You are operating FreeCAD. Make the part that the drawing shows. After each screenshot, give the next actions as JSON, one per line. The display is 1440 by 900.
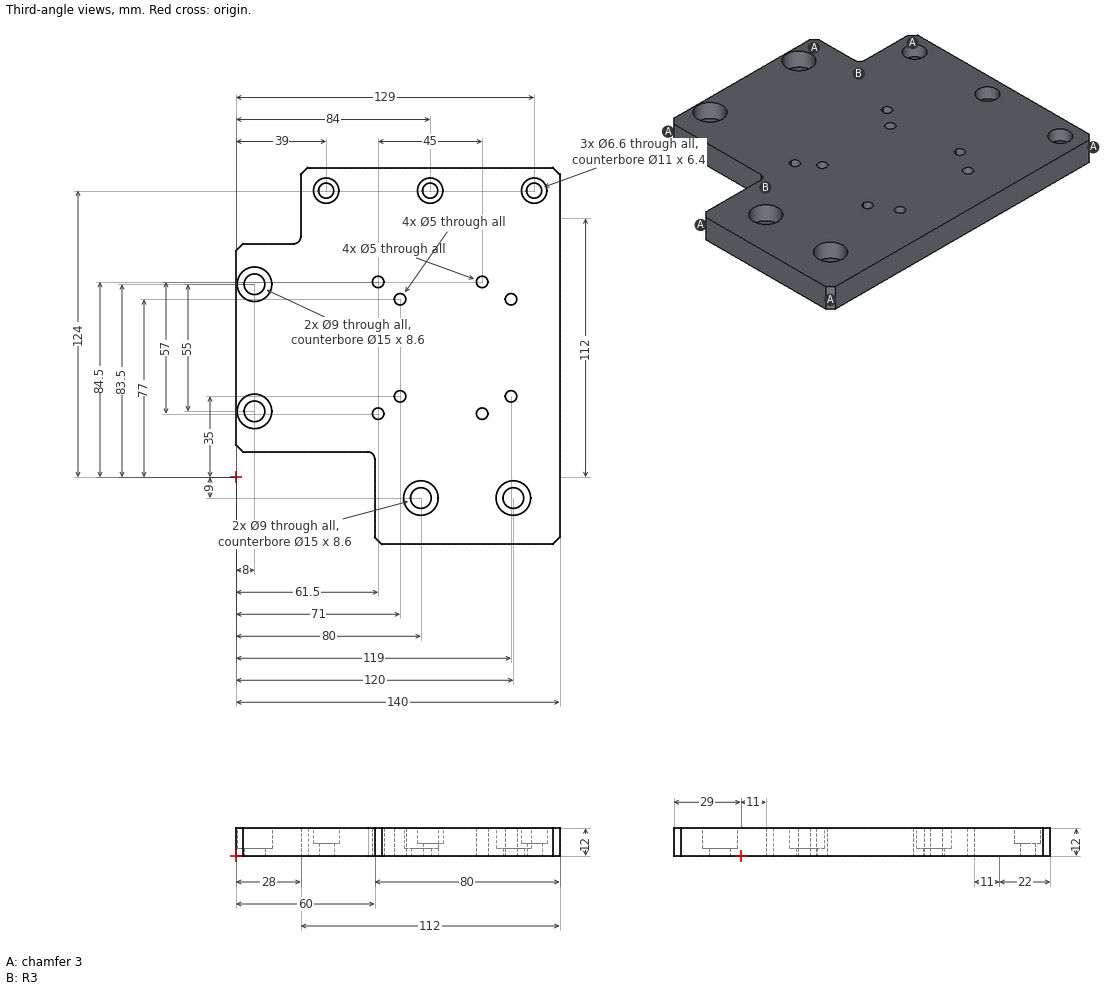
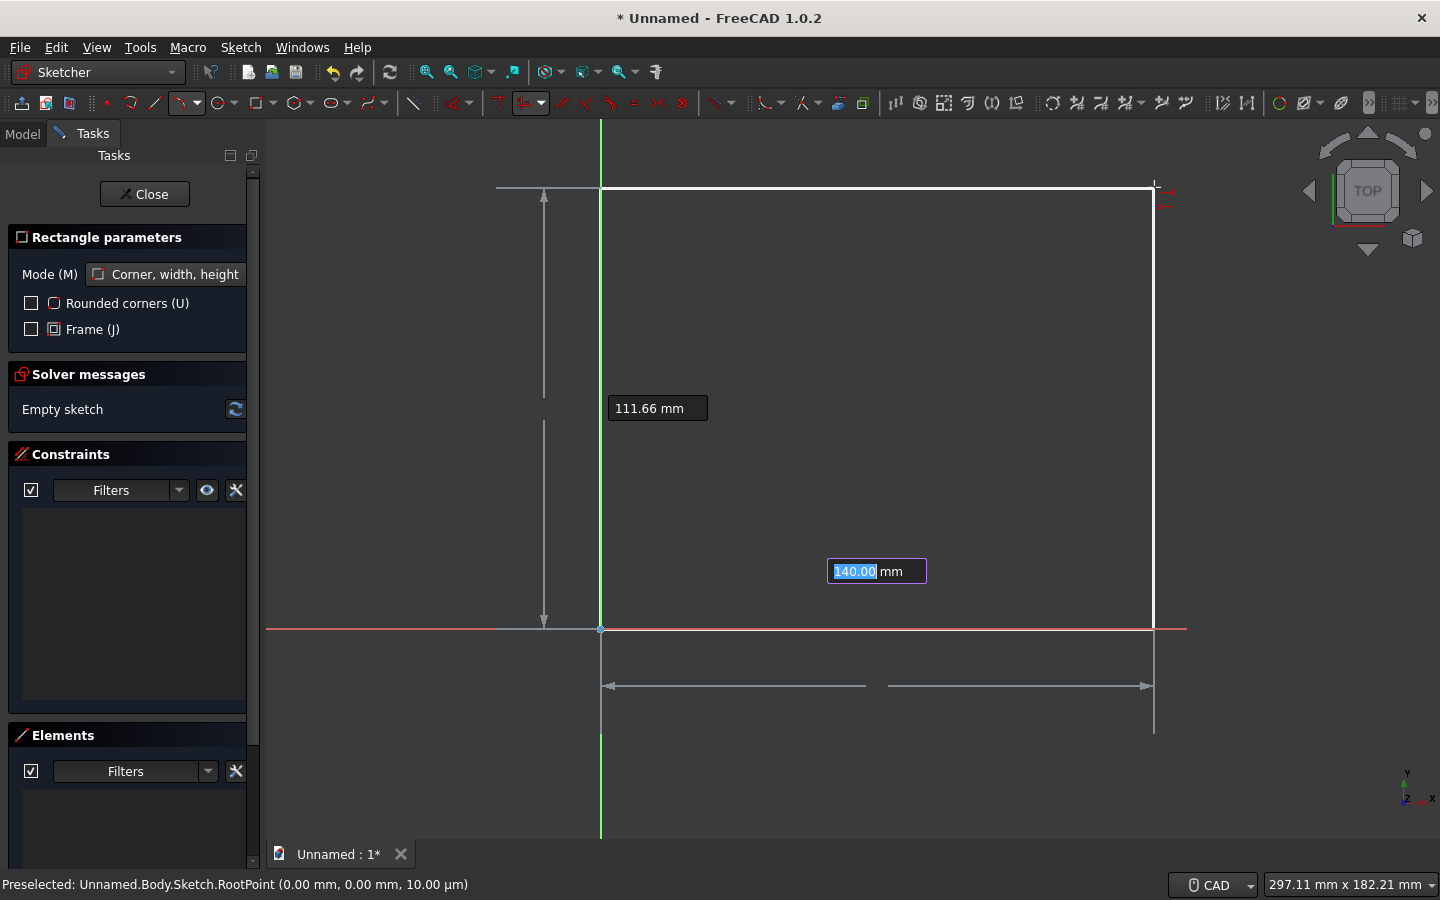
{"action": "type", "text": "140"}
{"action": "key", "text": "Tab"}
{"action": "type", "text": "112"}
{"action": "key", "text": "Return"}
{"action": "key", "text": "Escape"}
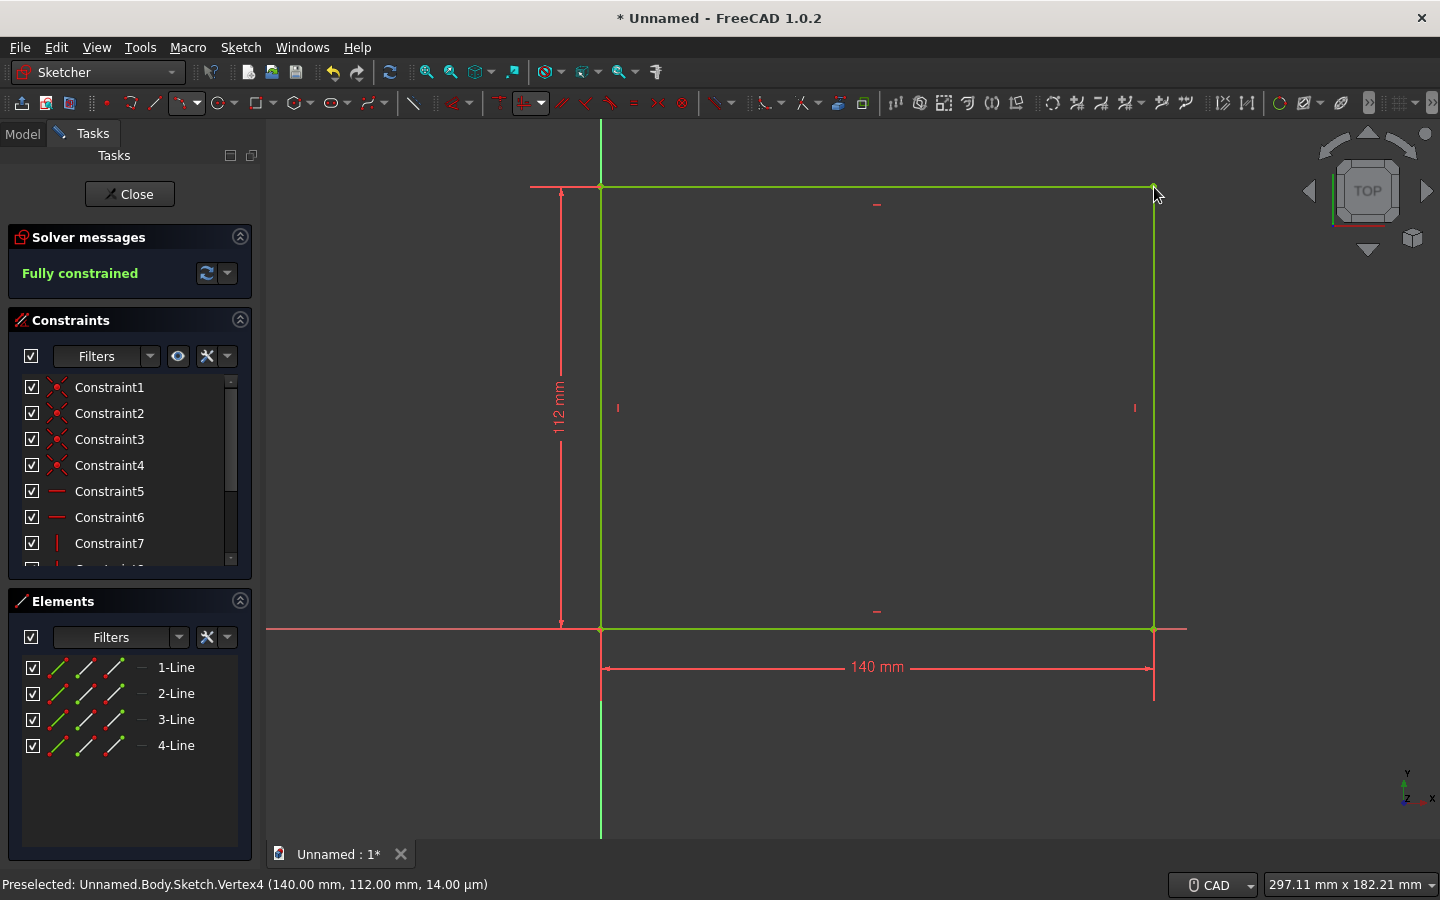
{"action": "left_click", "coordinate": [130, 194]}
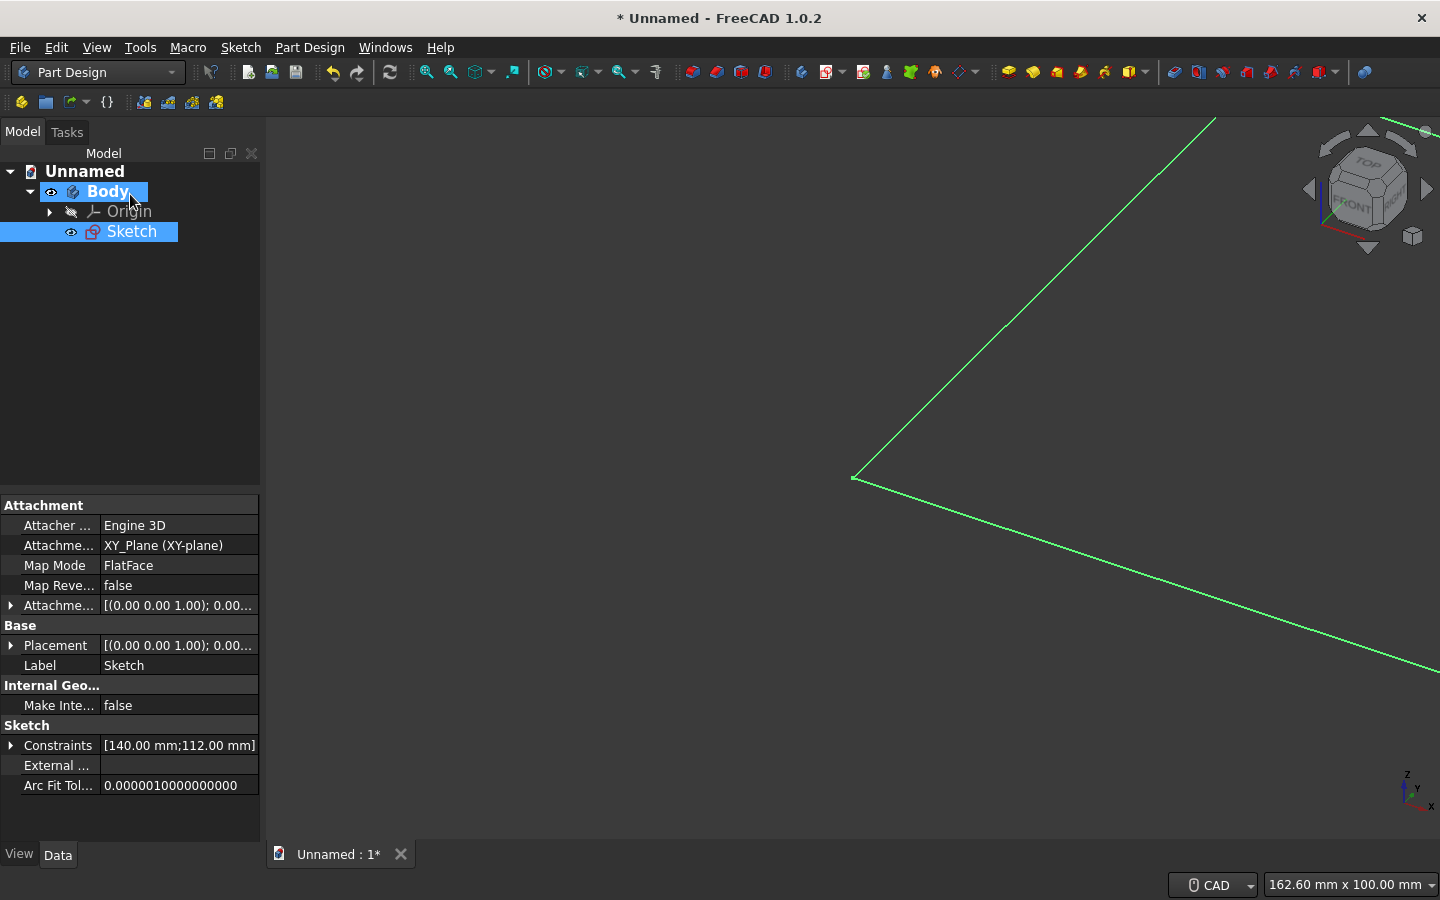
{"action": "left_click", "coordinate": [1010, 72]}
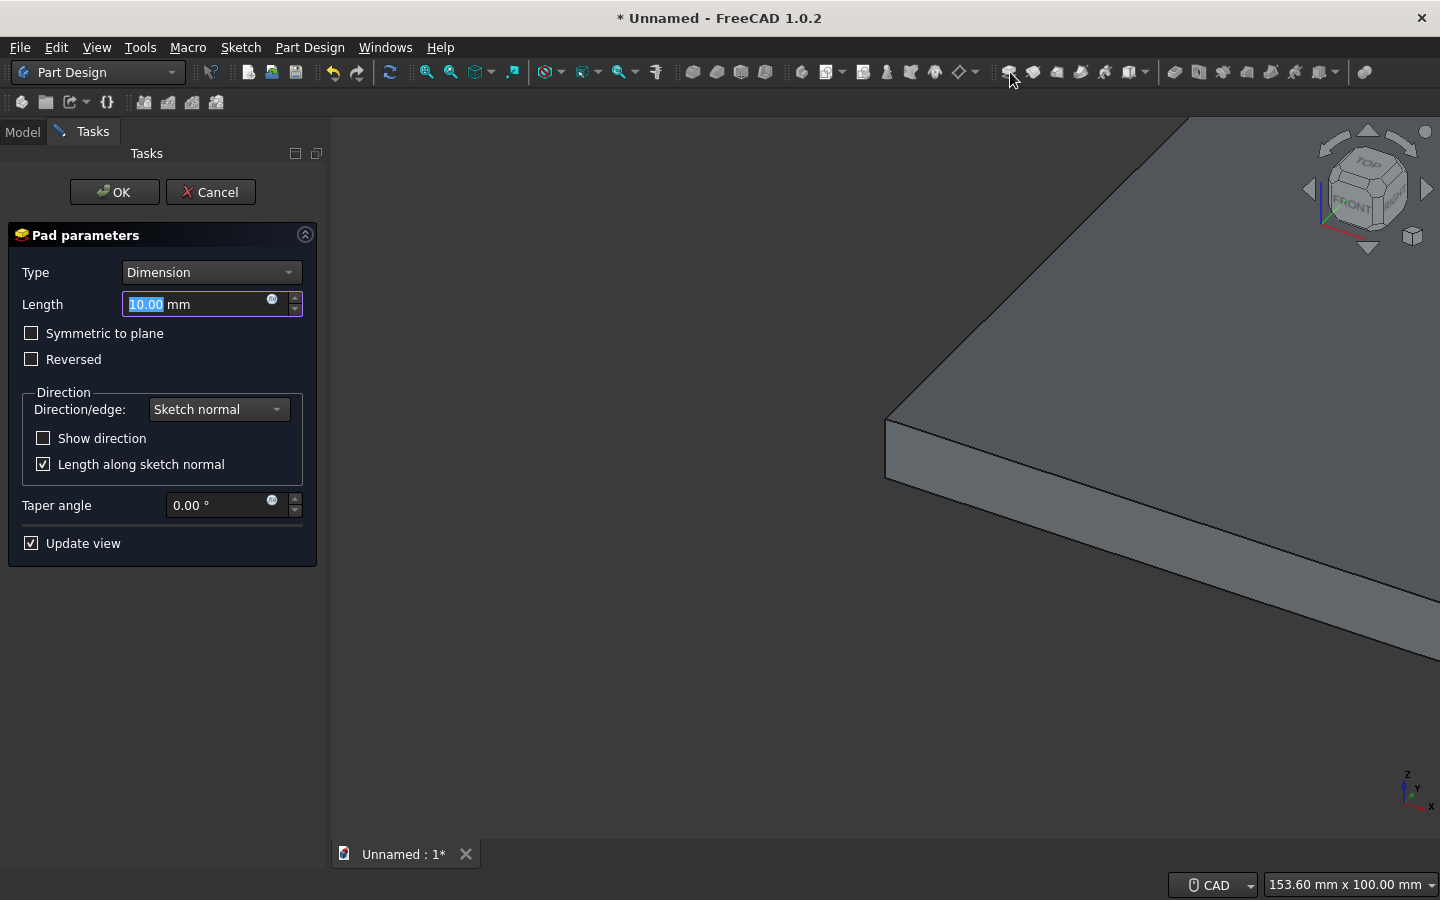
{"action": "type", "text": "12"}
{"action": "key", "text": "Tab"}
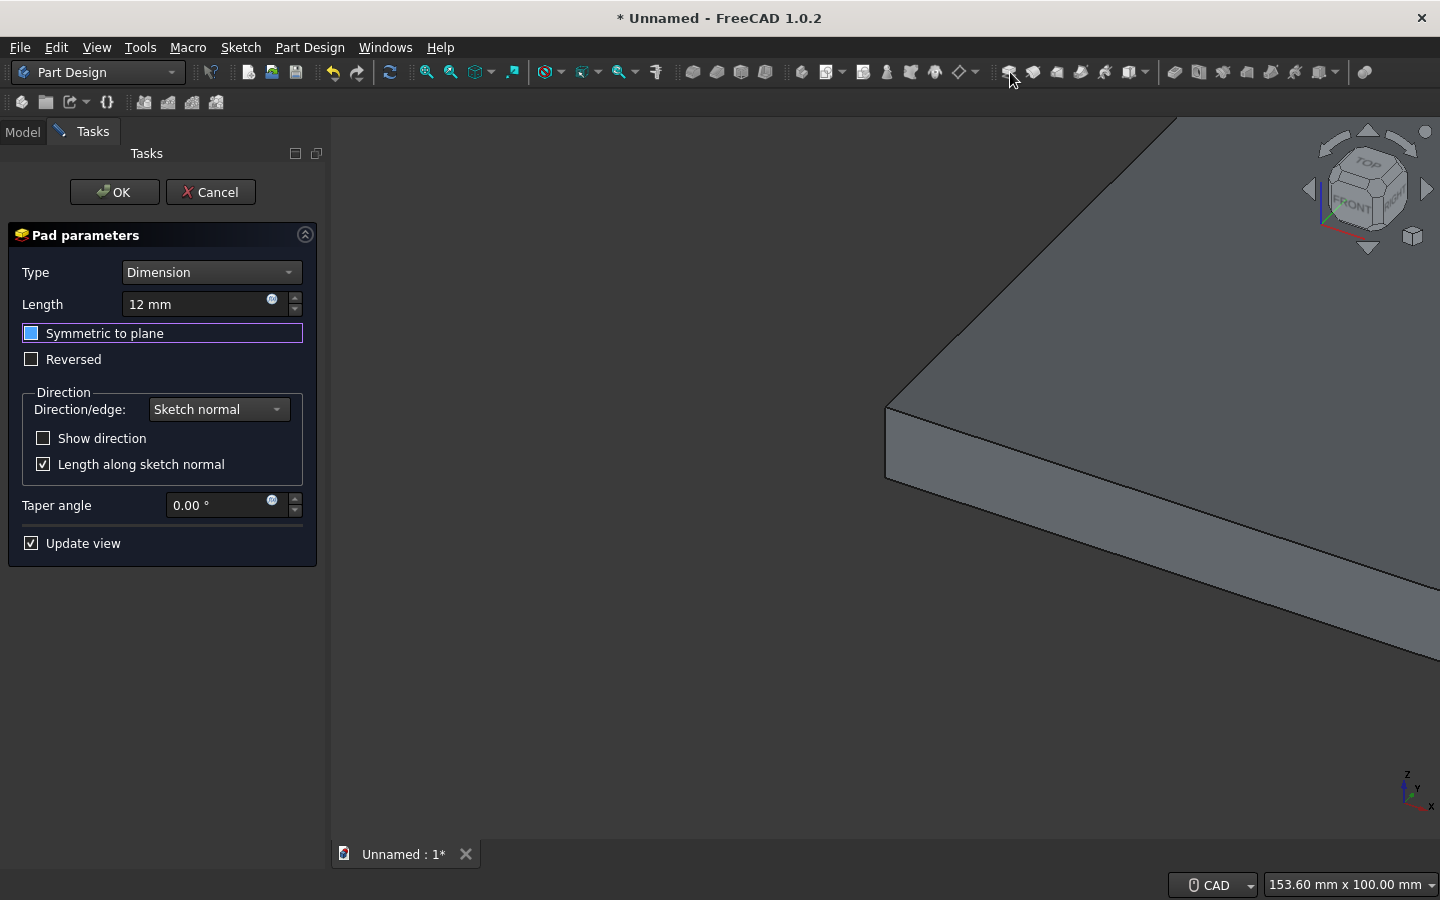
{"action": "left_click", "coordinate": [115, 192]}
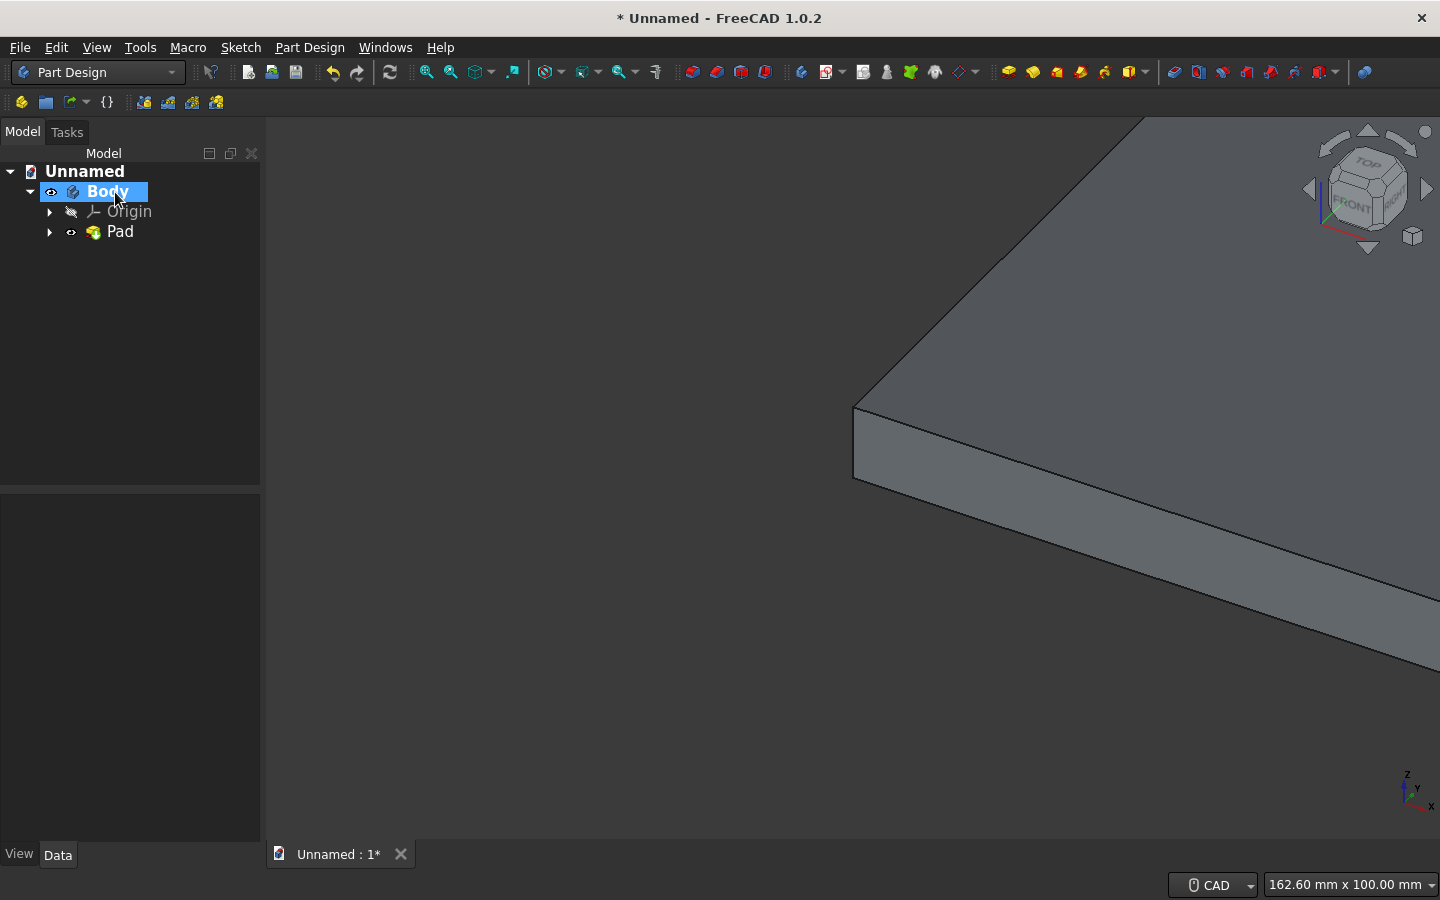
{"action": "left_click", "coordinate": [428, 72]}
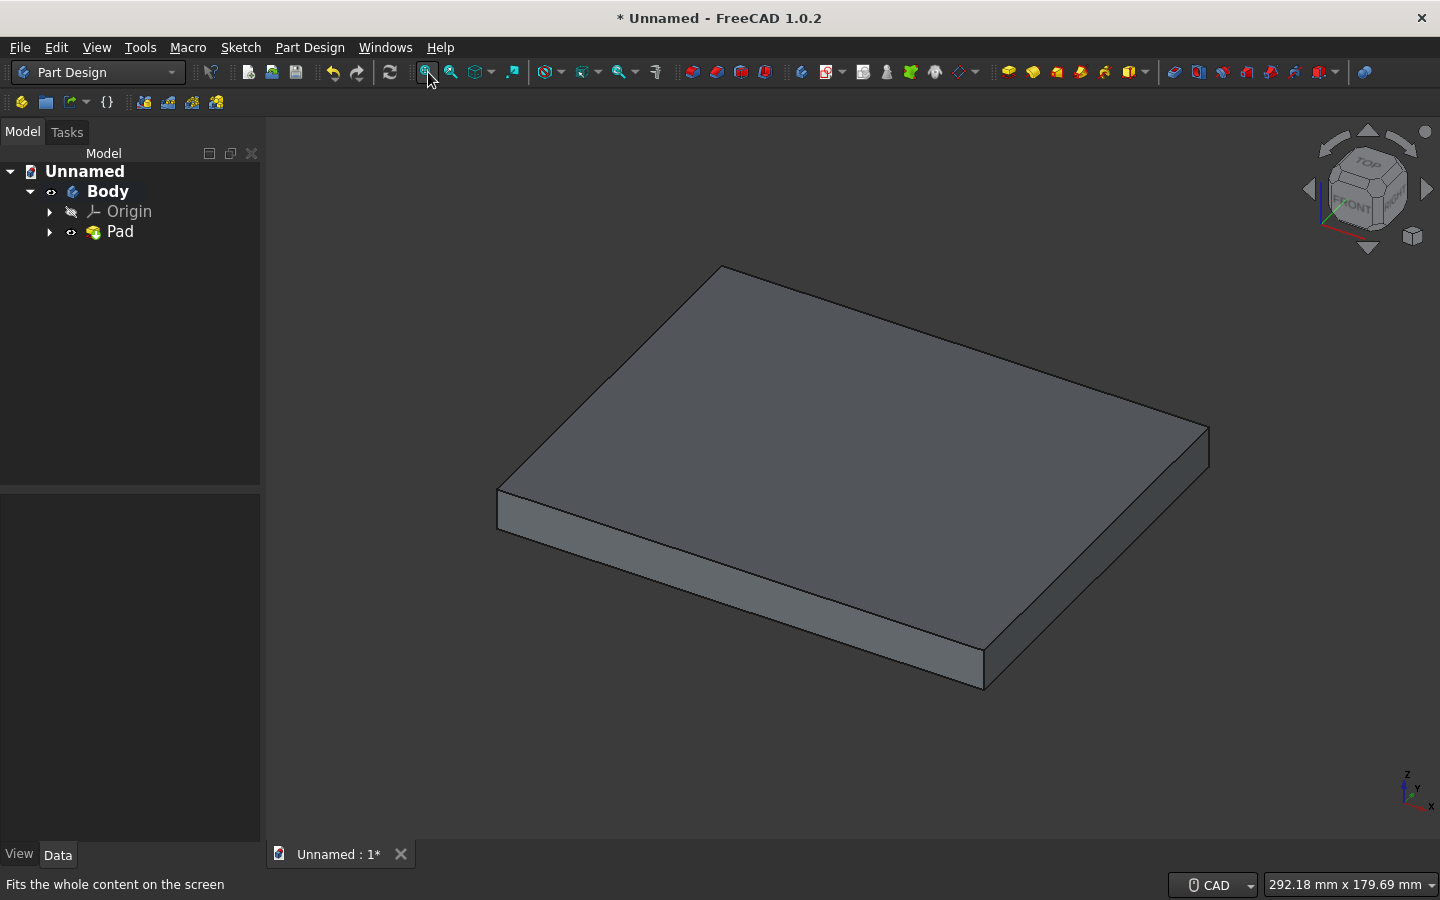
{"action": "key", "text": "5"}